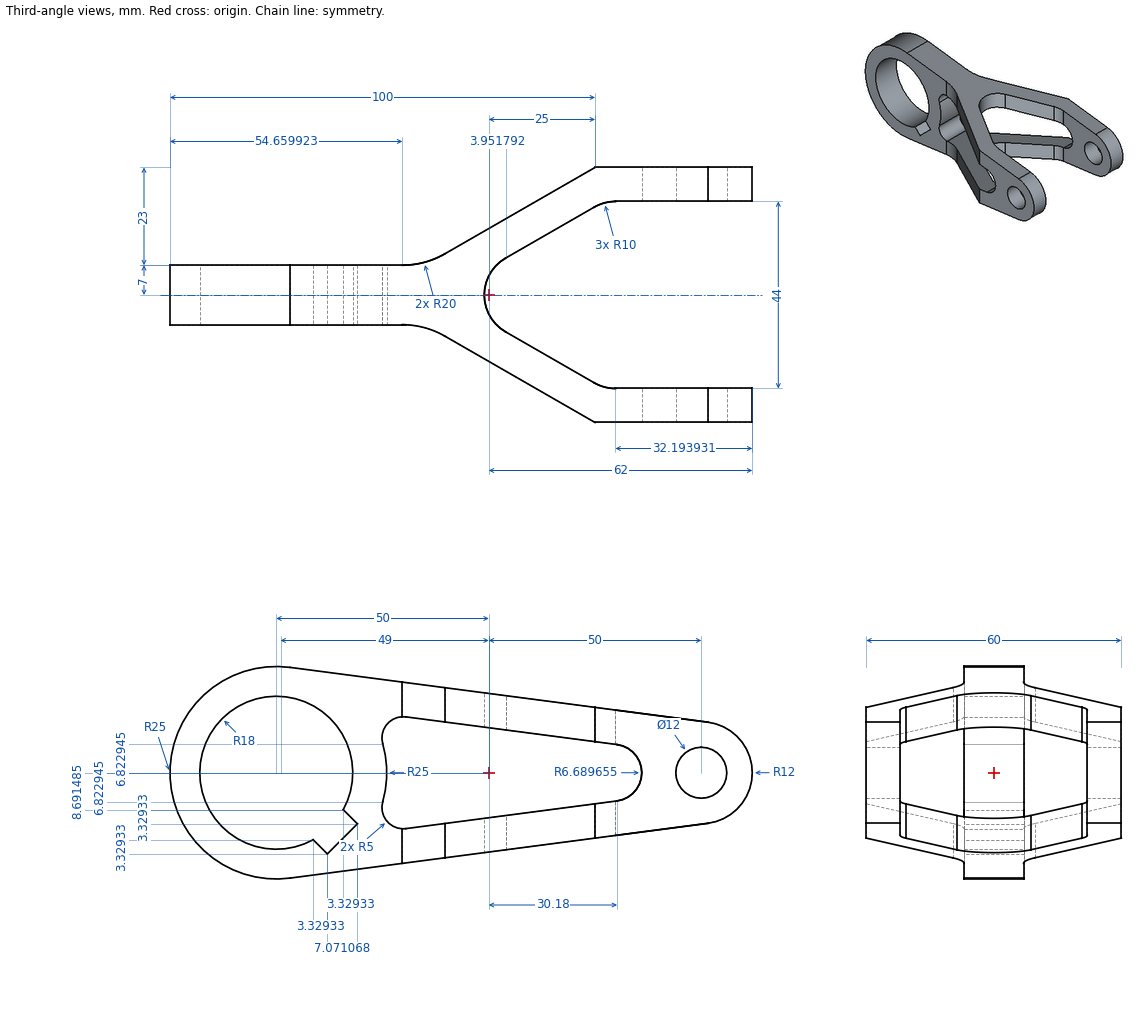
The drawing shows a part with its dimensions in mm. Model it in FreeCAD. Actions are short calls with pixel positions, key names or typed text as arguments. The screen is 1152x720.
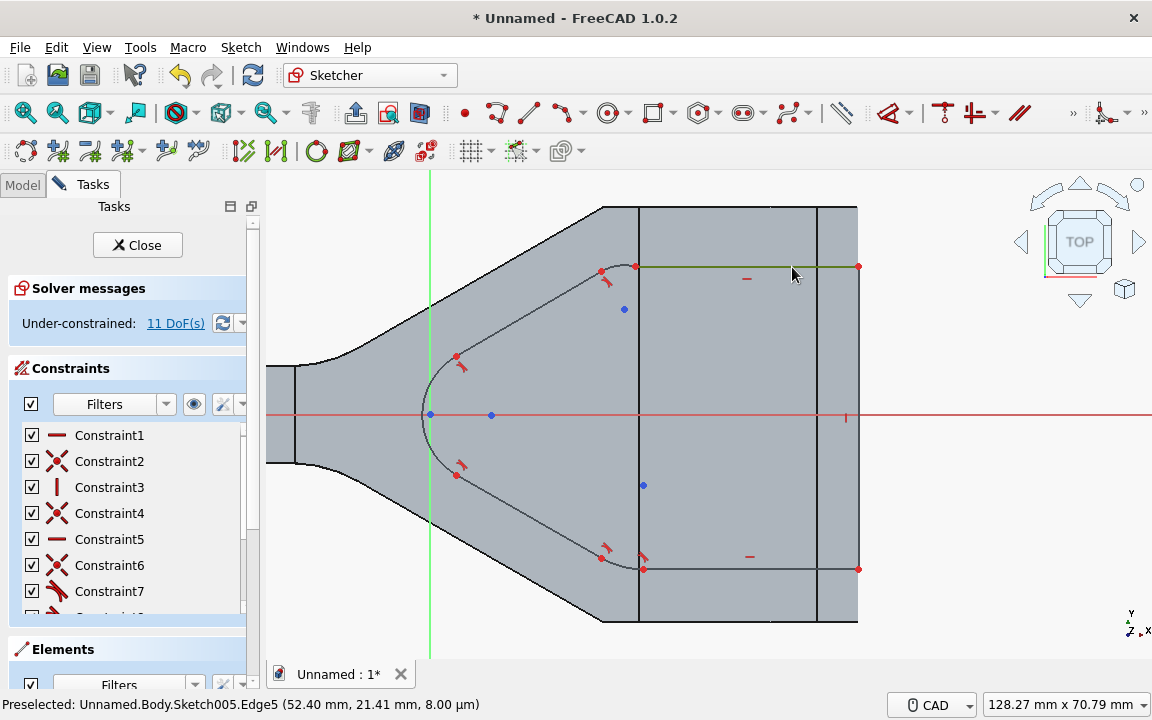
scroll(625, 265, up, 2)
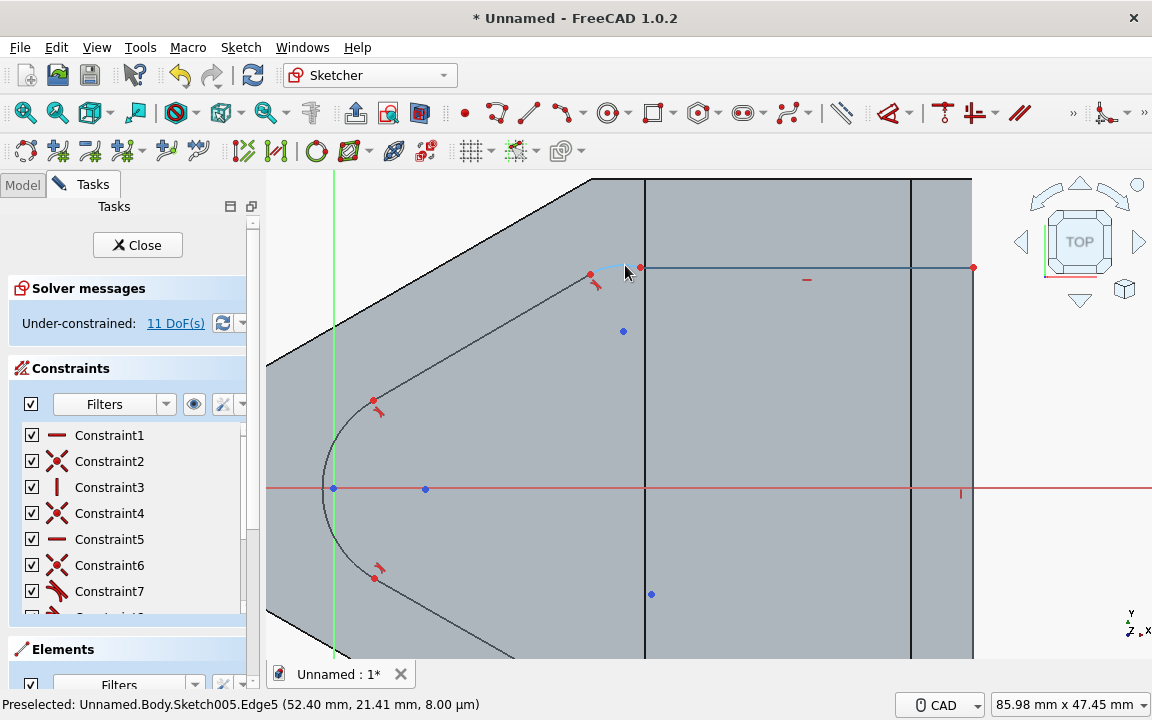
click(625, 265)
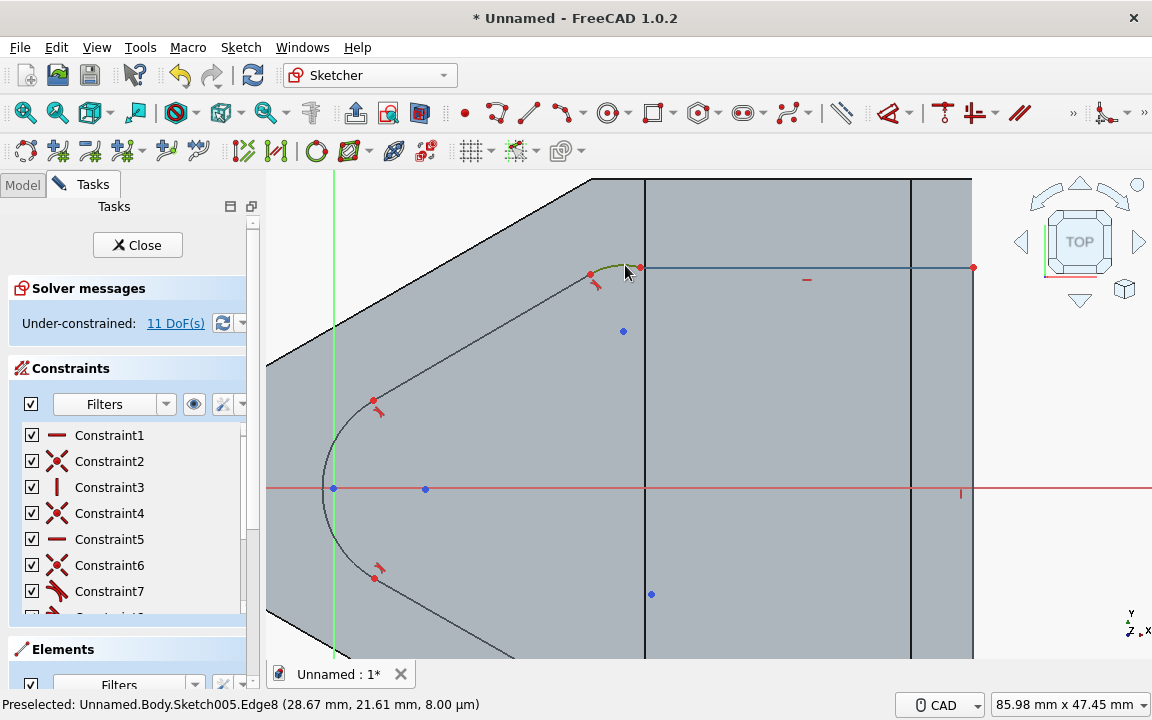
key(t)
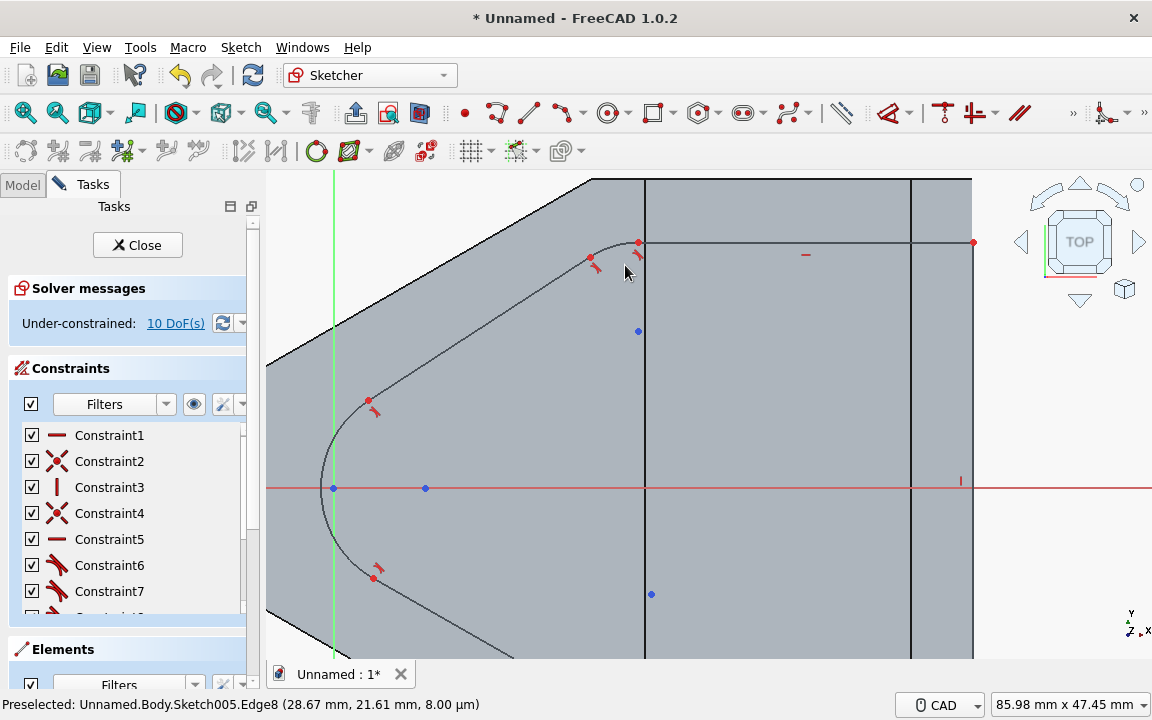
click(331, 532)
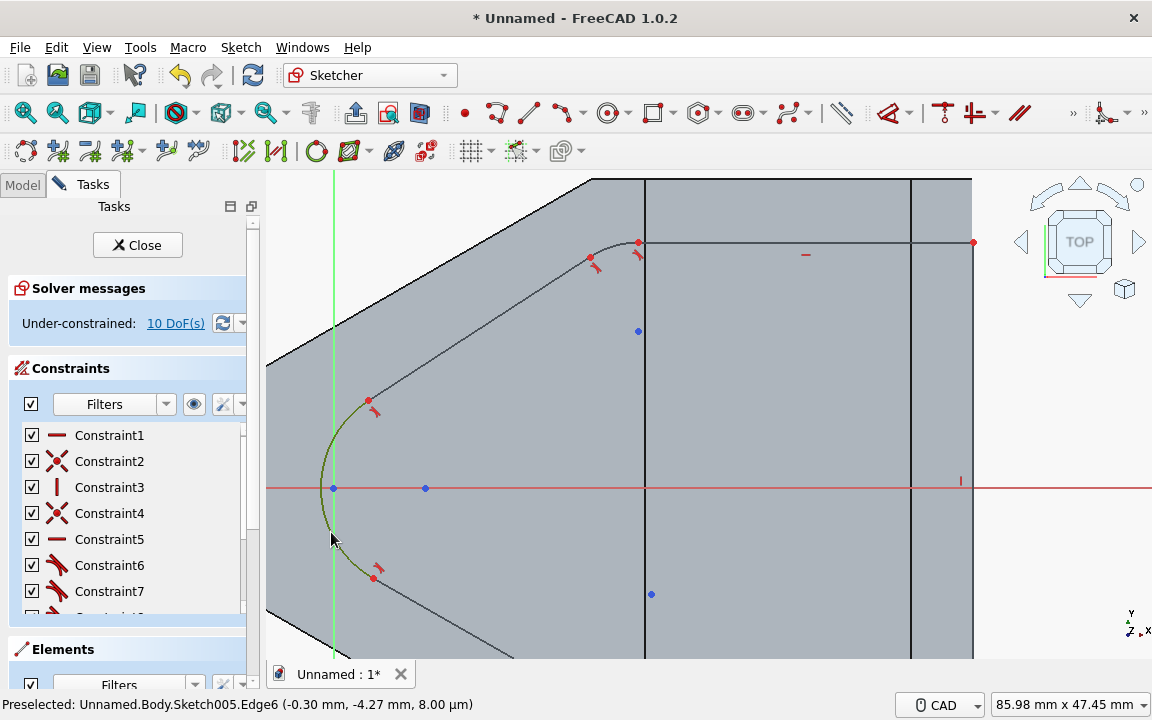
scroll(625, 265, down, 2)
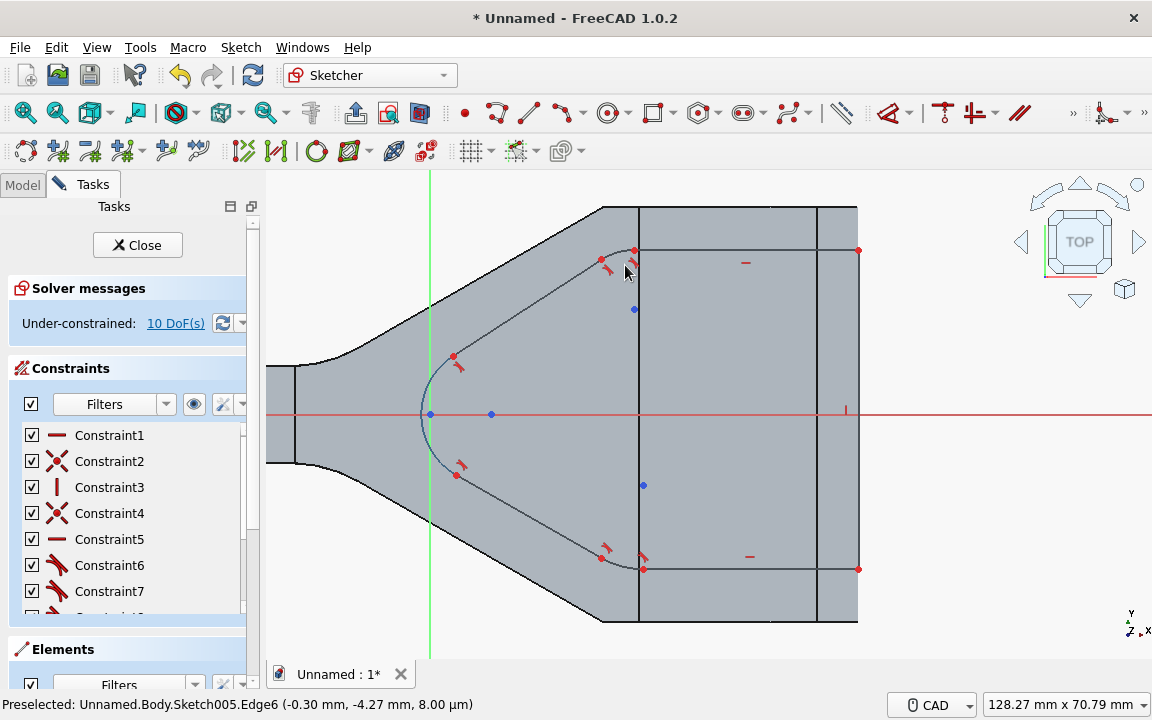
click(613, 564)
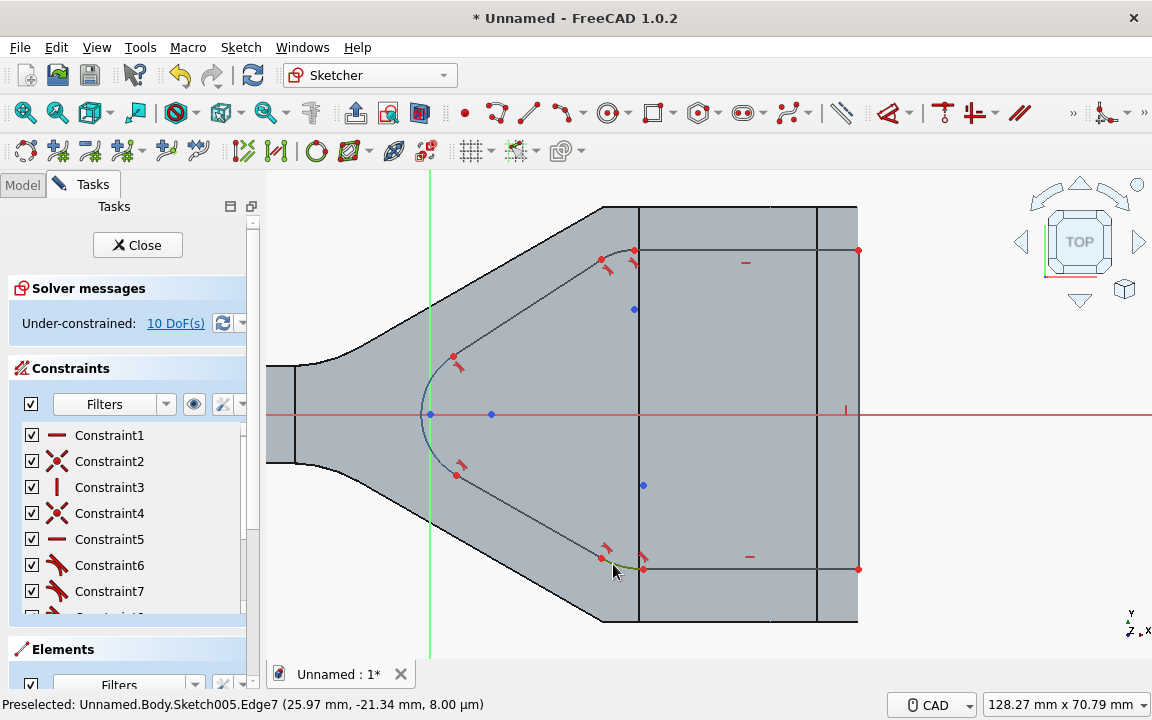
scroll(624, 251, up, 2)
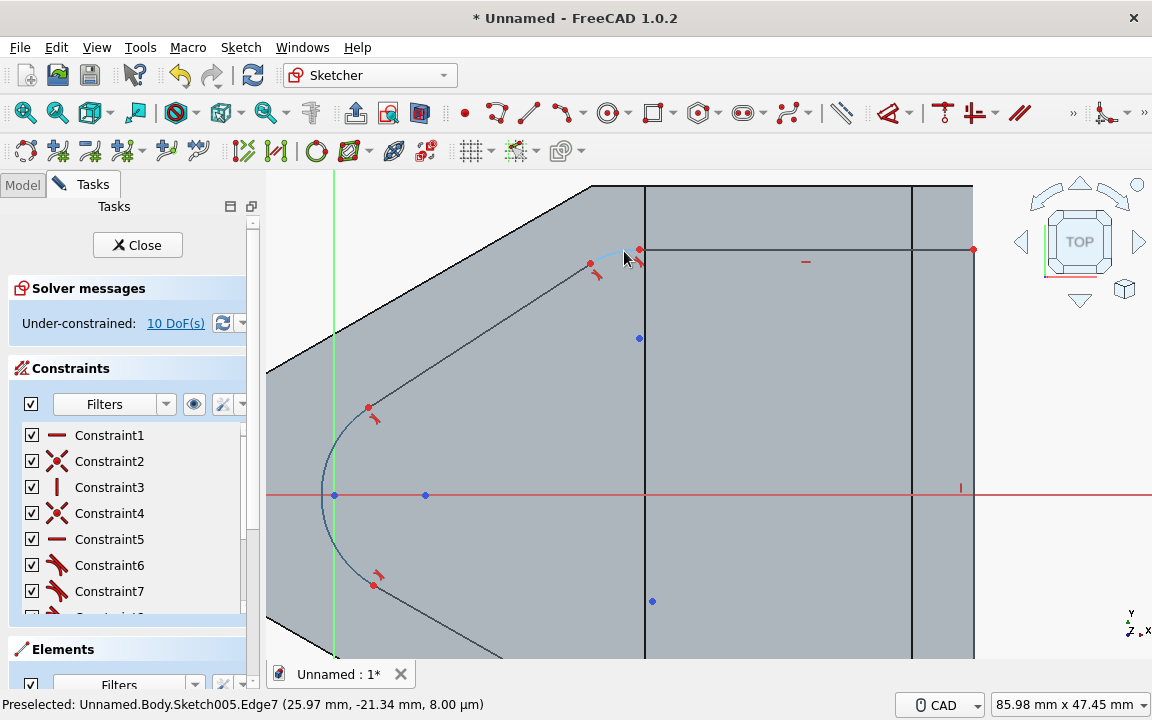
click(624, 251)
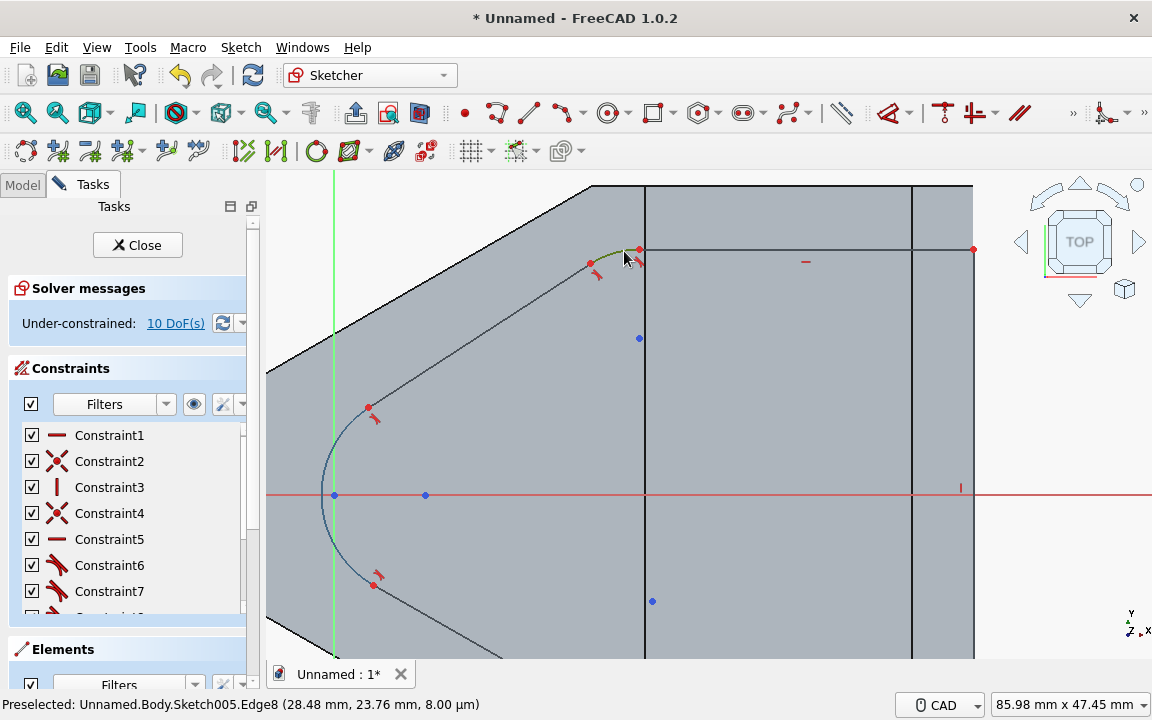
key(e)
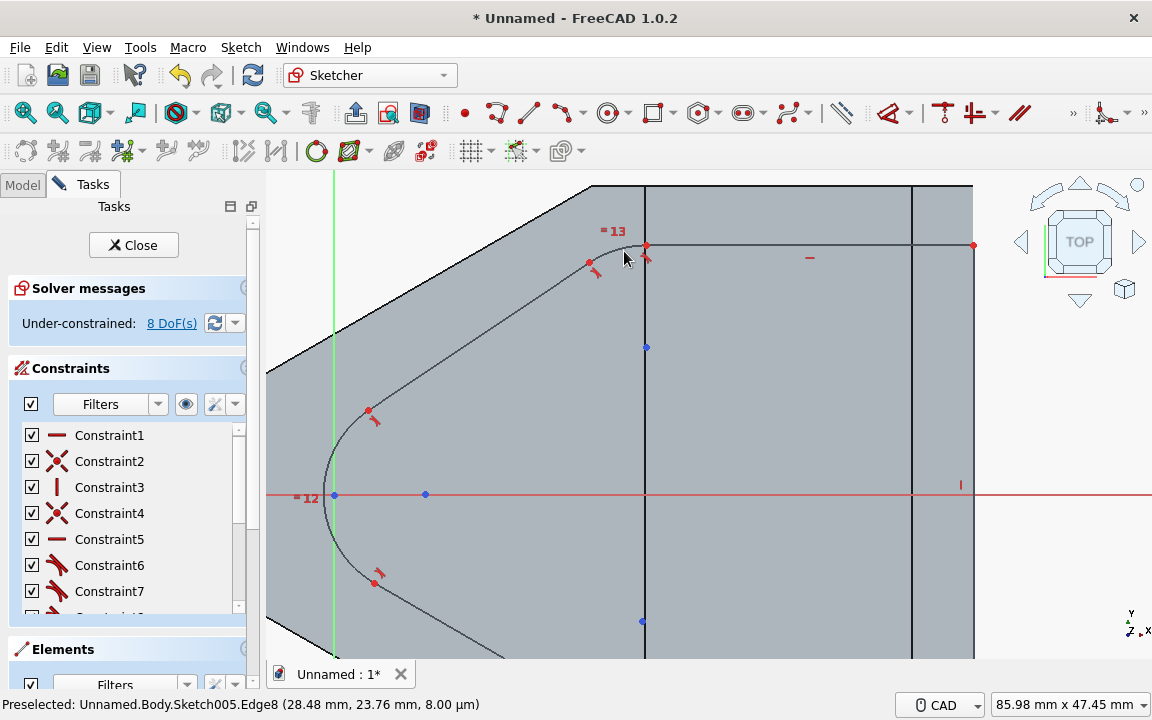
click(426, 495)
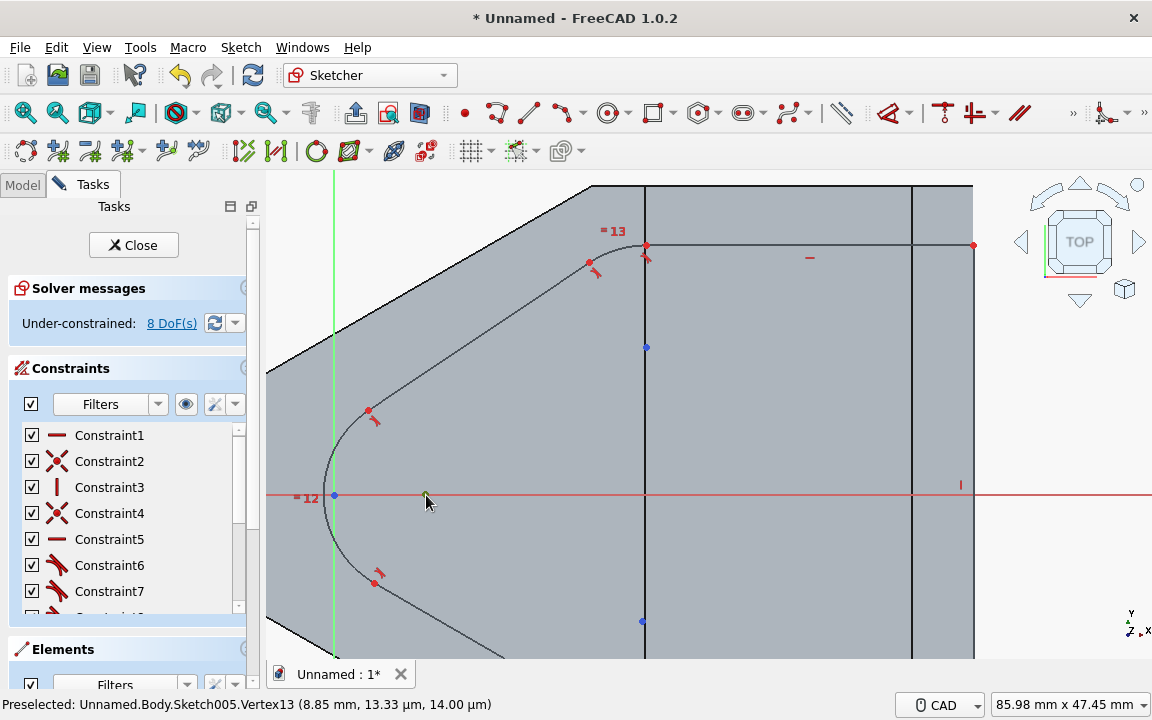
click(393, 495)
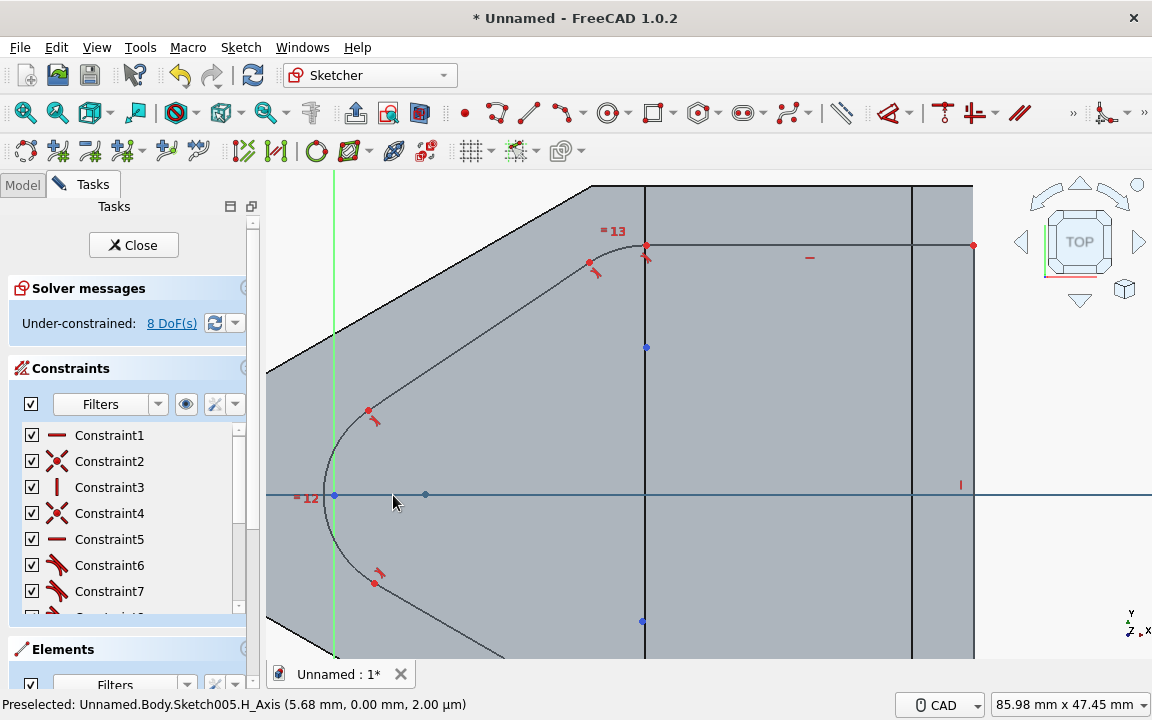
key(c)